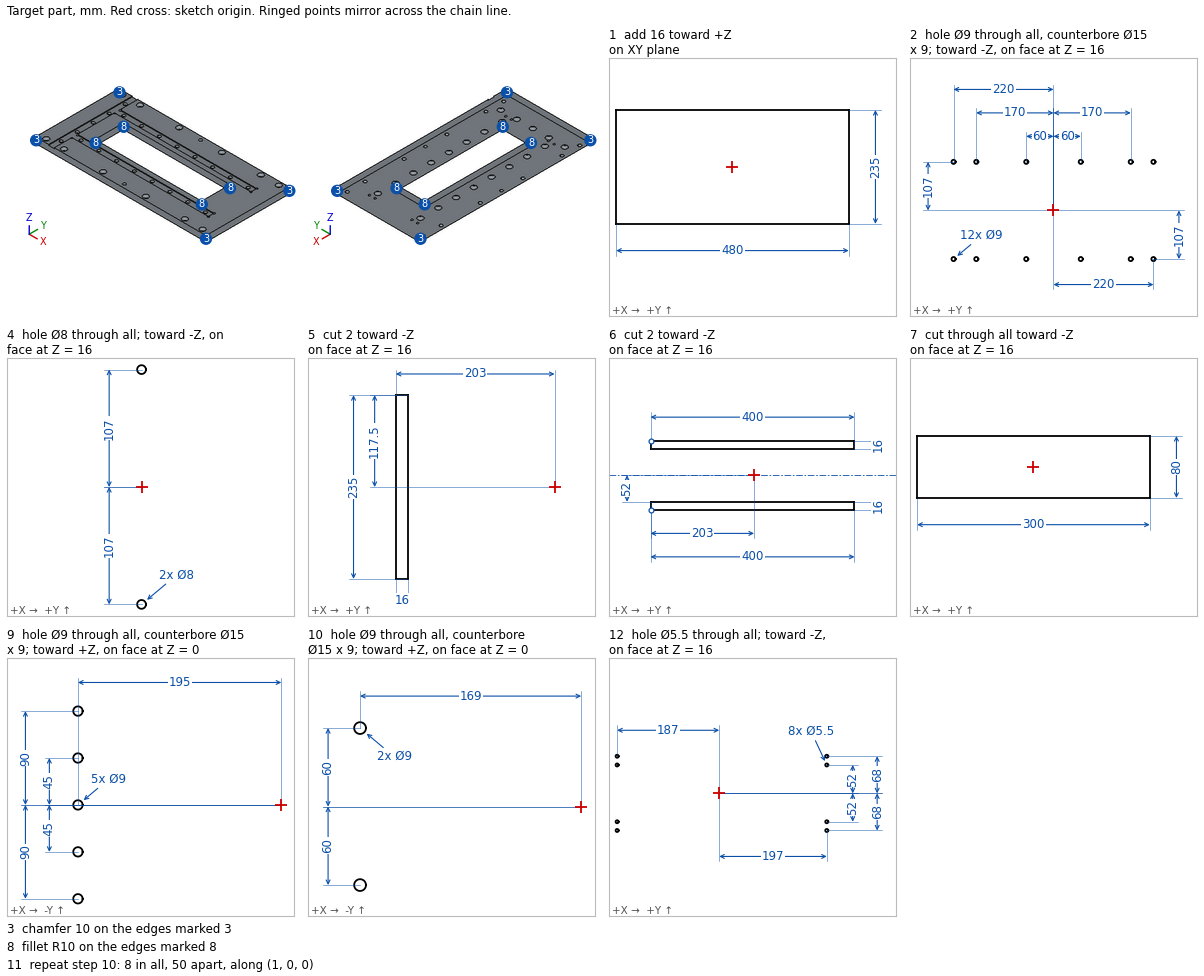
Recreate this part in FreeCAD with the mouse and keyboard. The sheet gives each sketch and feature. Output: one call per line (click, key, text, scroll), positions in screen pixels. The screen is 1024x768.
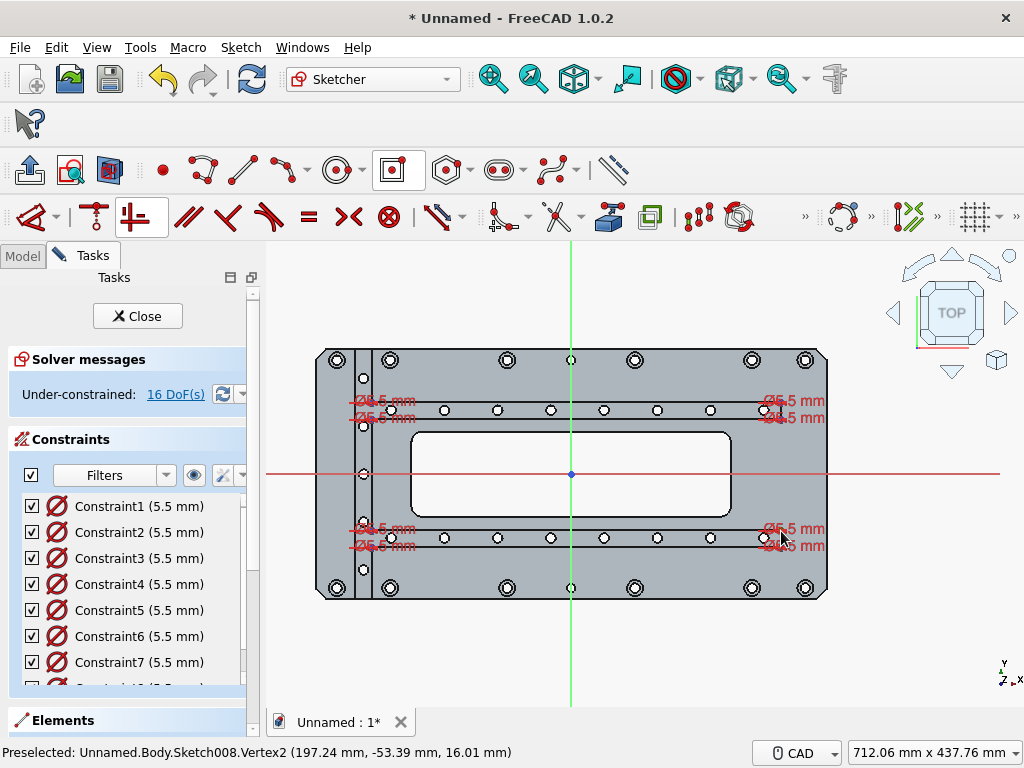
click(162, 218)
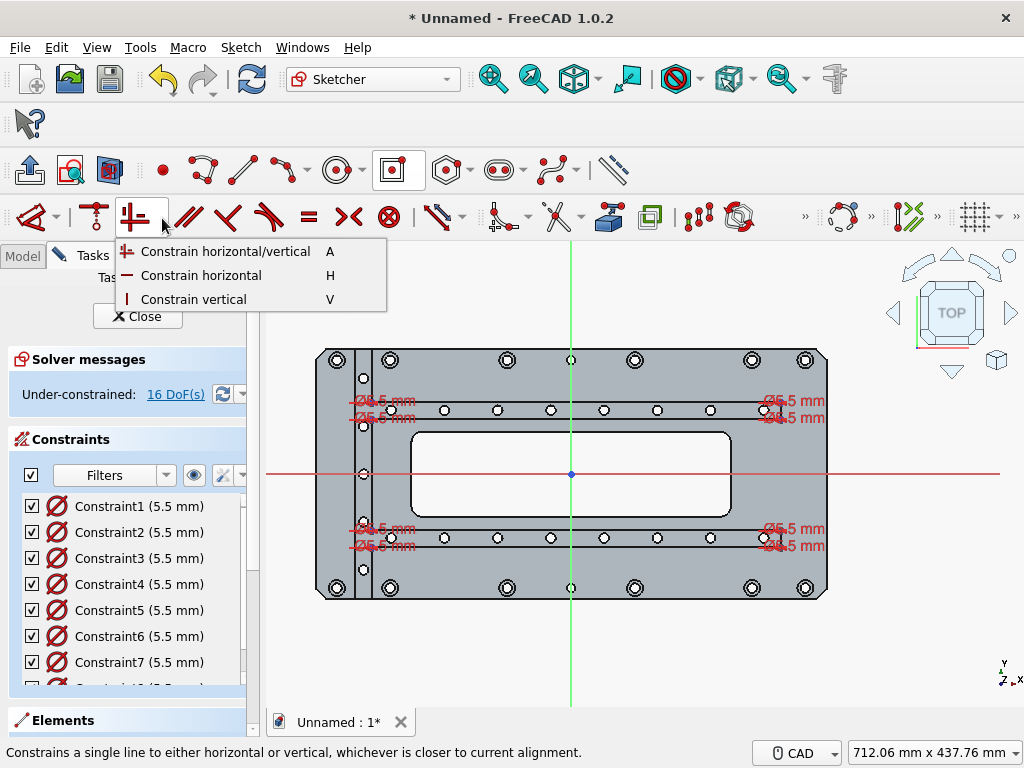
click(251, 299)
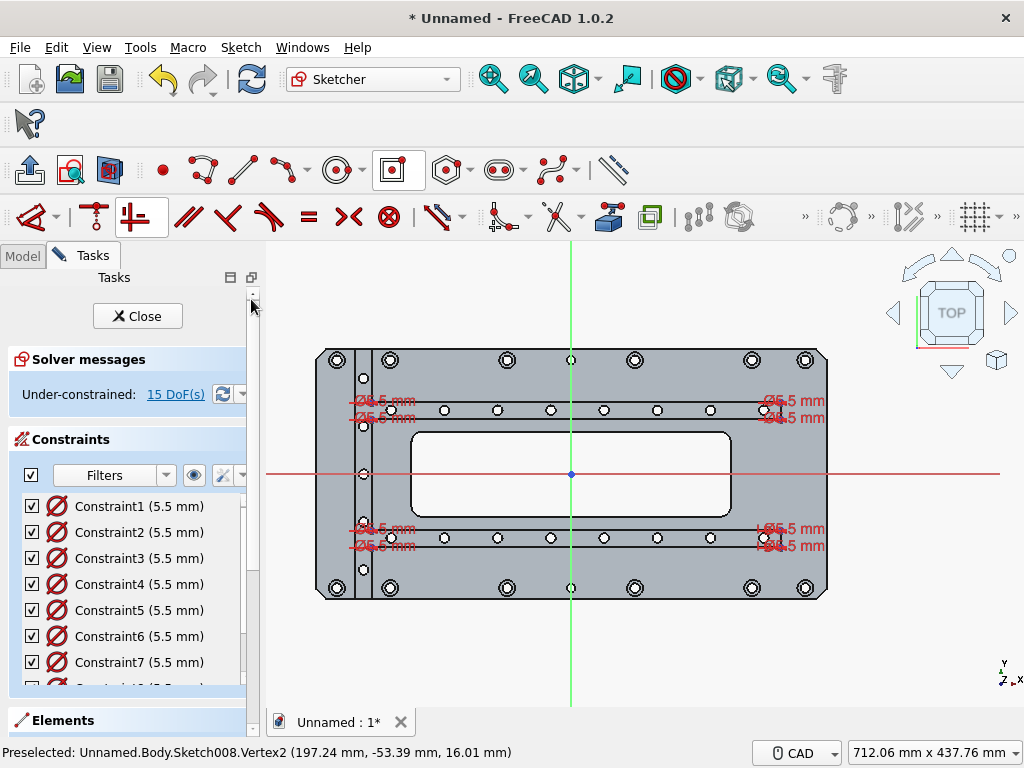
click(781, 531)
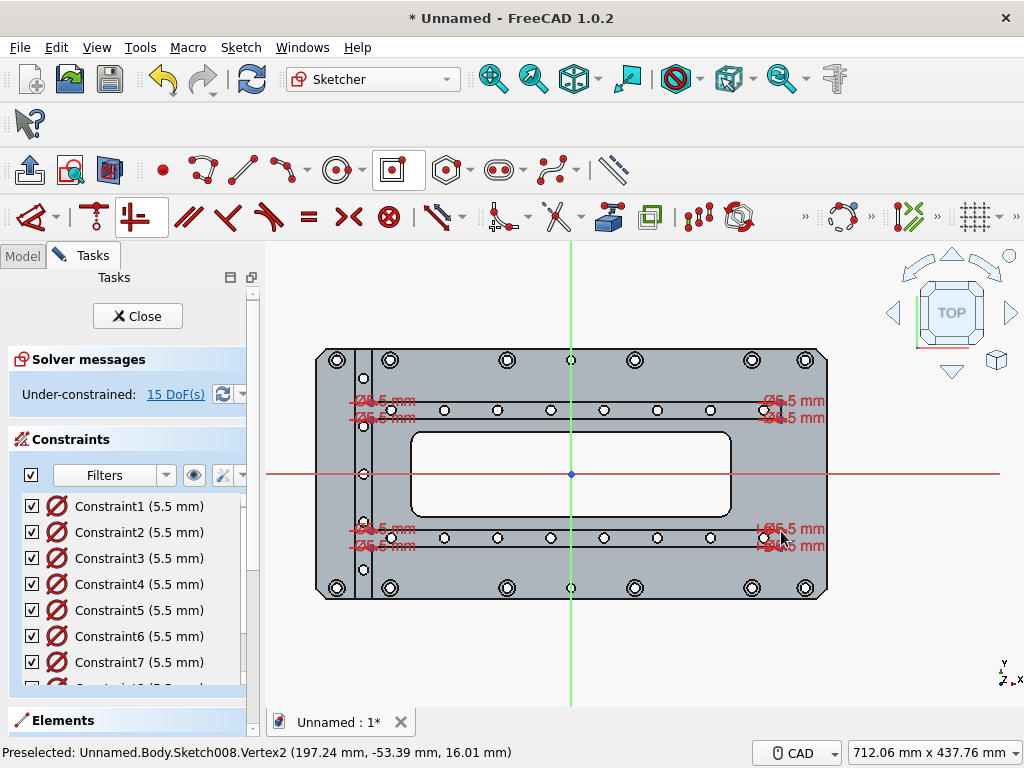
click(781, 420)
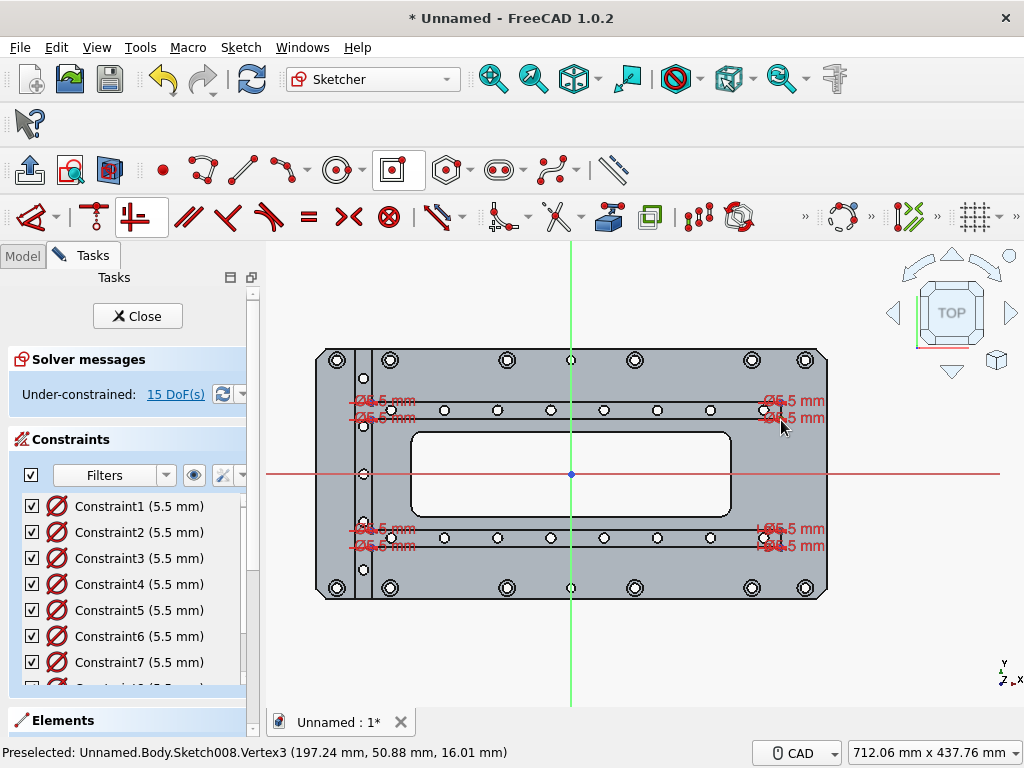
click(162, 218)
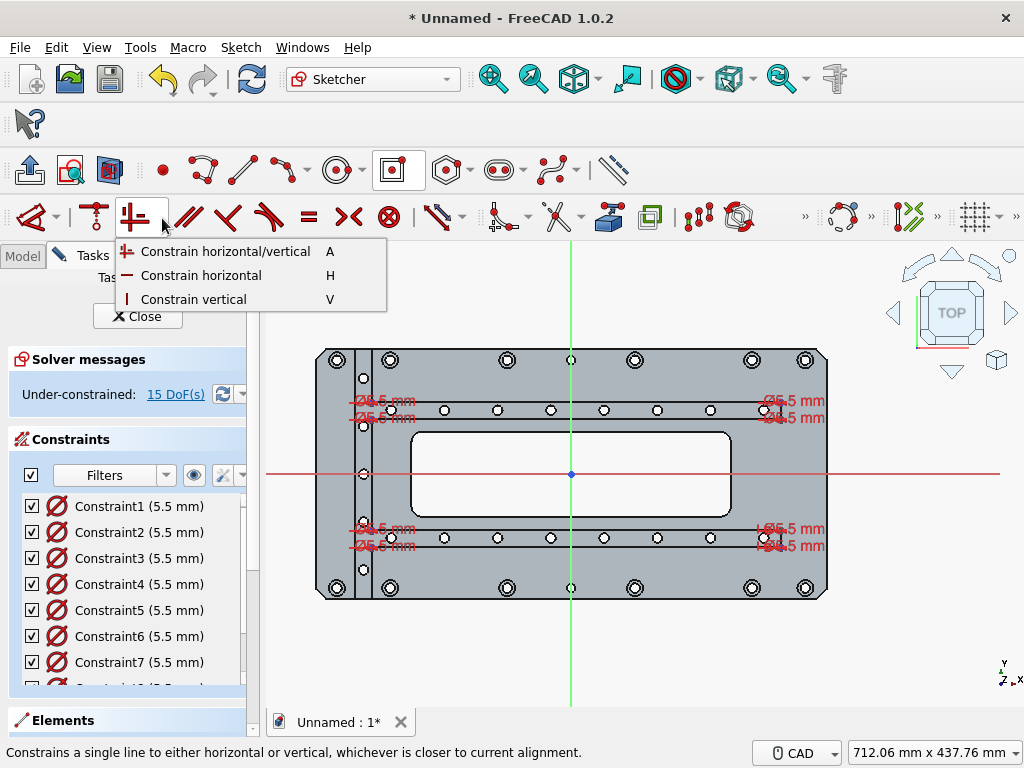
click(251, 299)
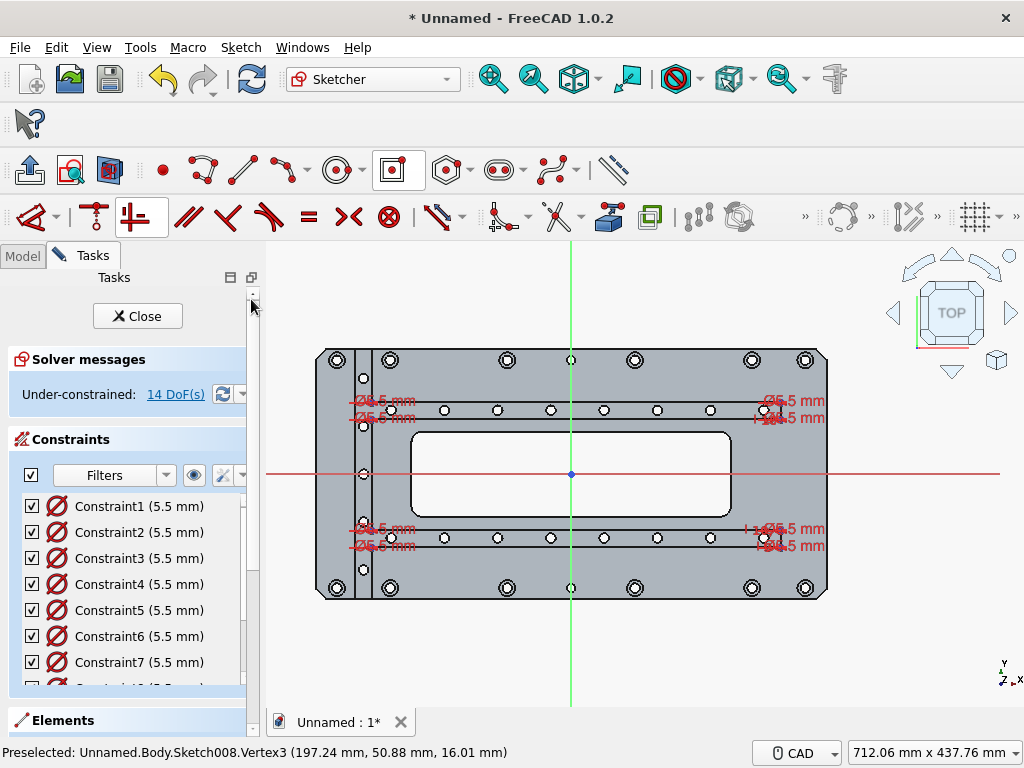
click(781, 420)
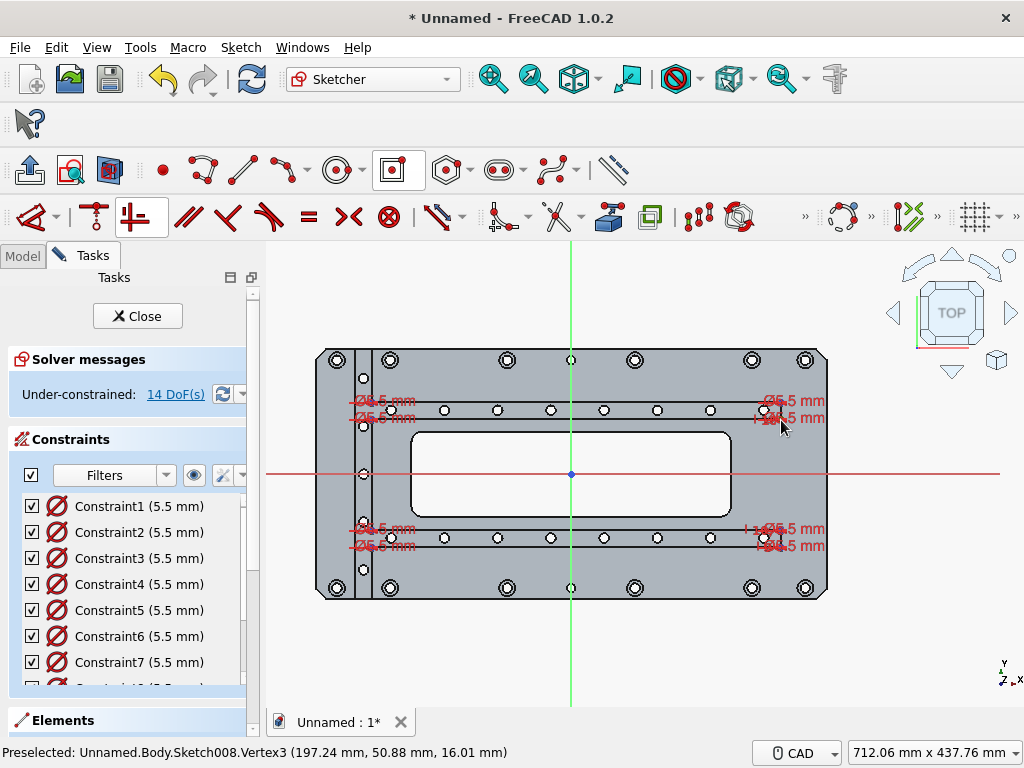
click(781, 403)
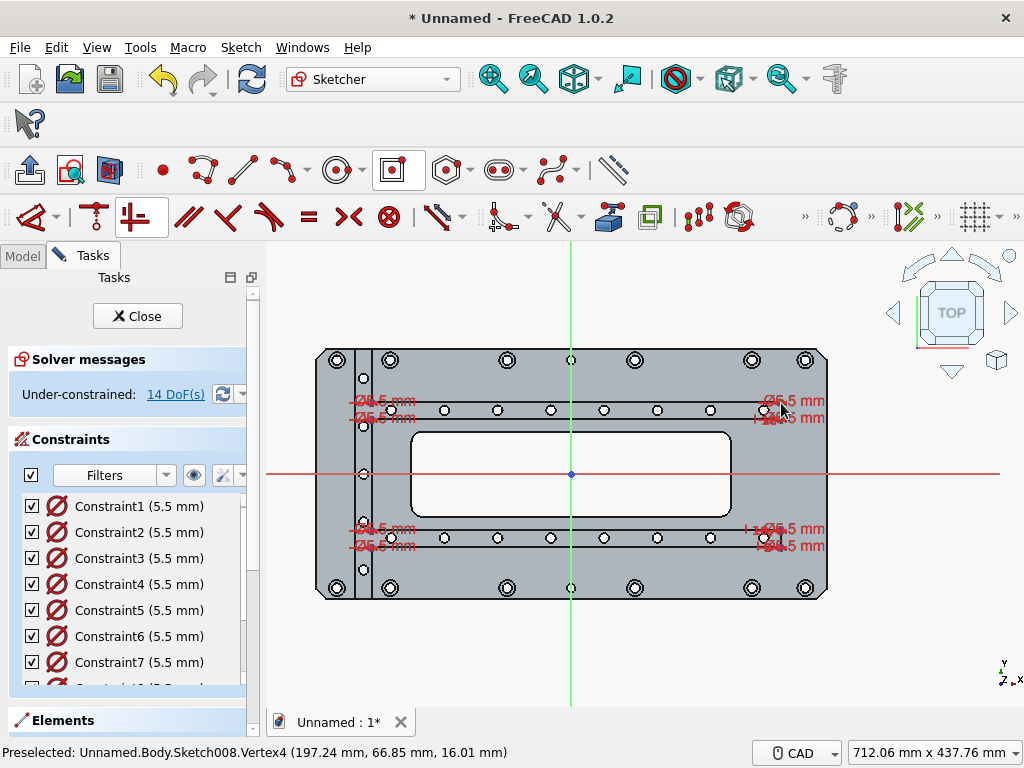
click(162, 218)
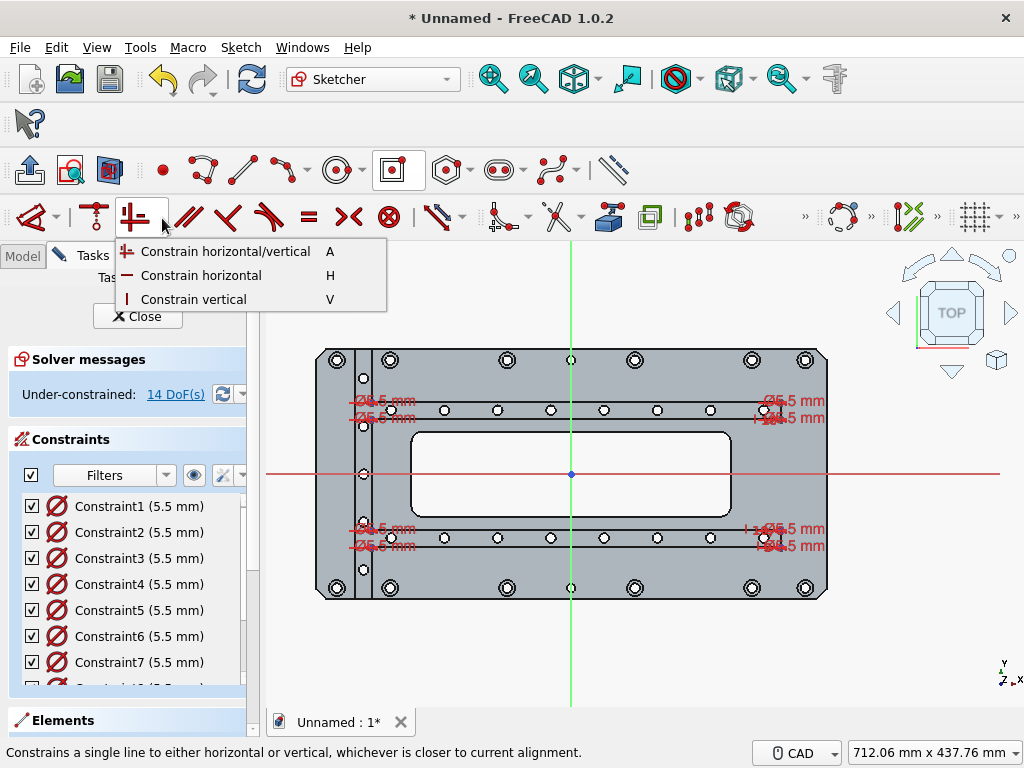
click(251, 299)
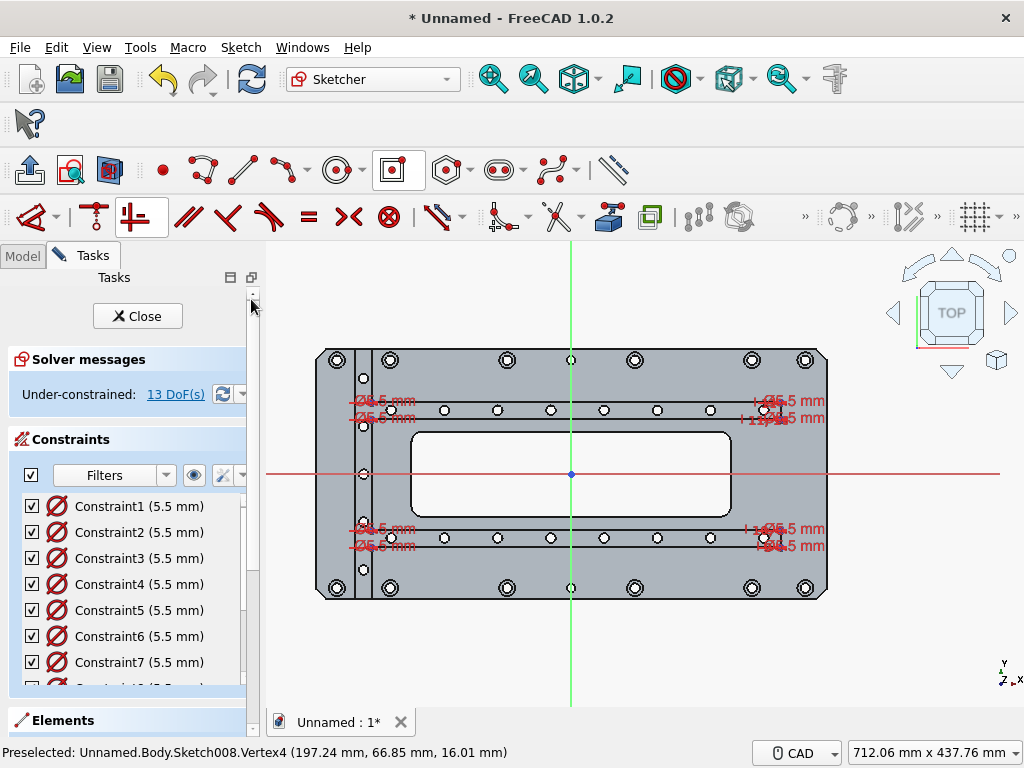
click(781, 403)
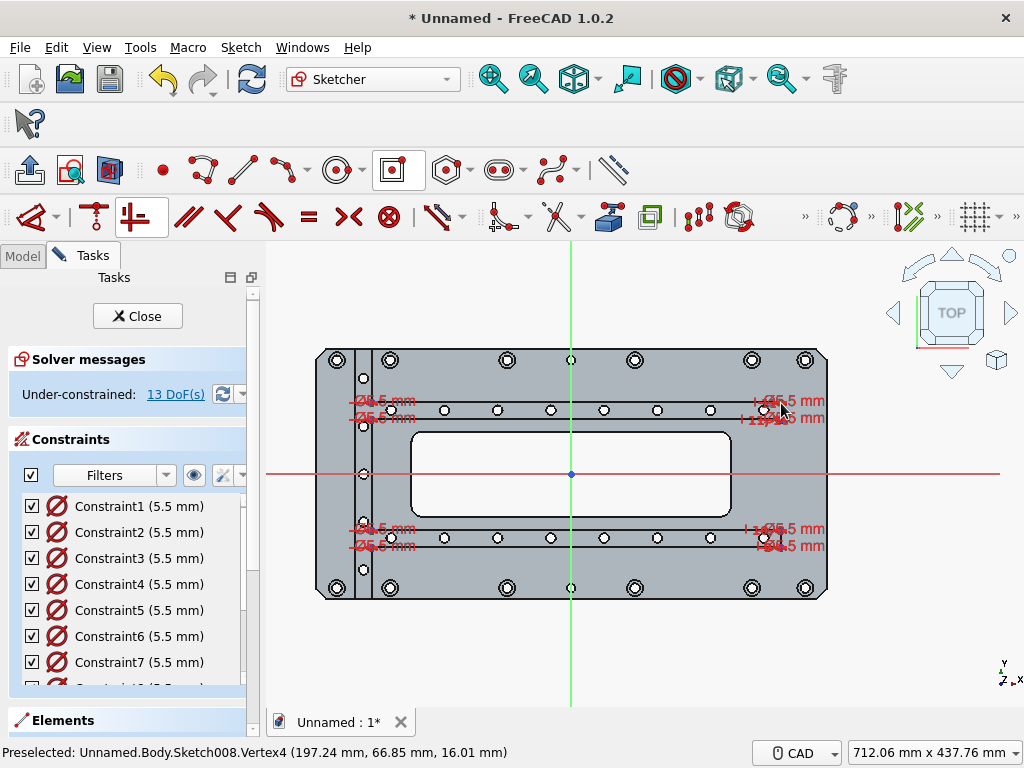
click(372, 403)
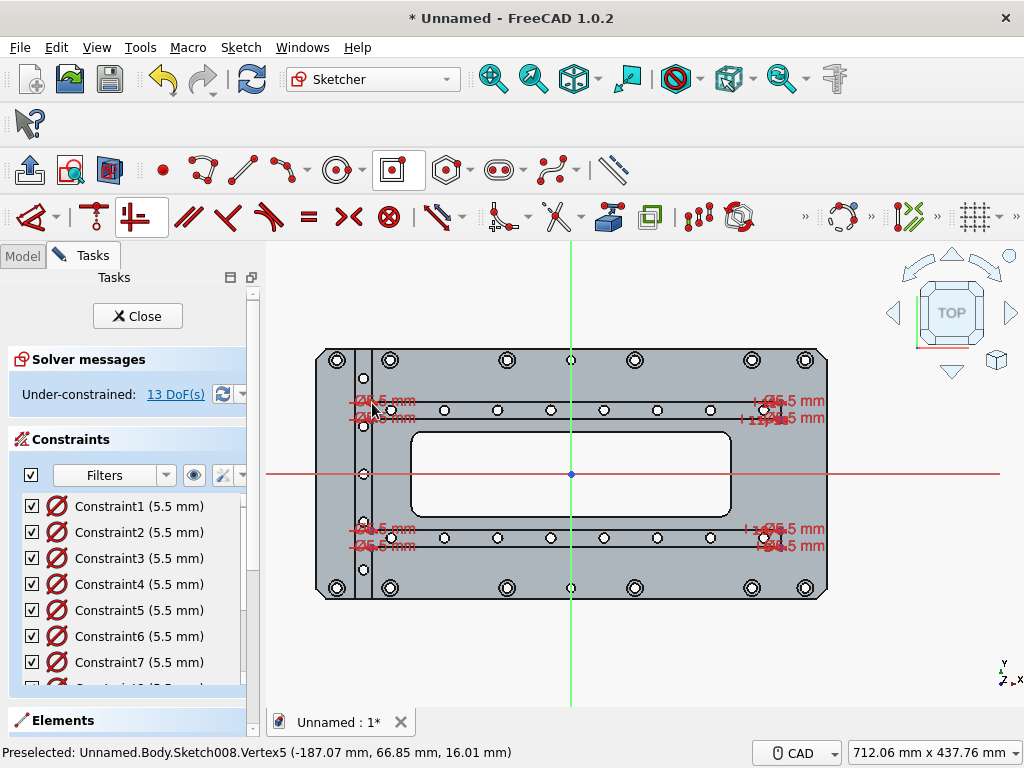
click(162, 218)